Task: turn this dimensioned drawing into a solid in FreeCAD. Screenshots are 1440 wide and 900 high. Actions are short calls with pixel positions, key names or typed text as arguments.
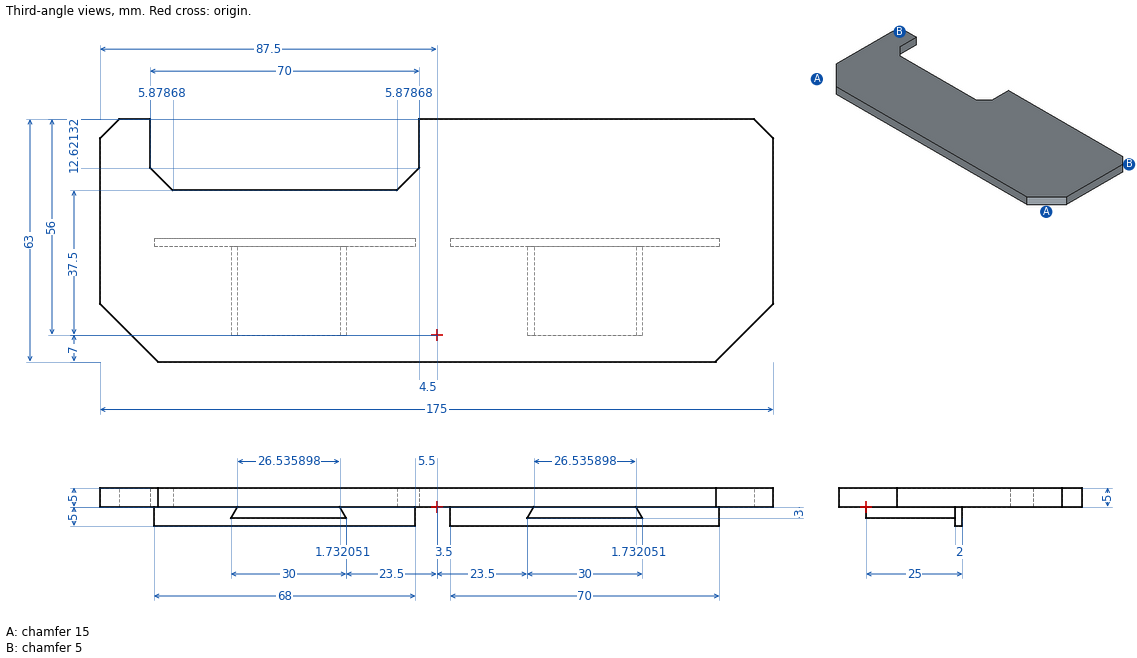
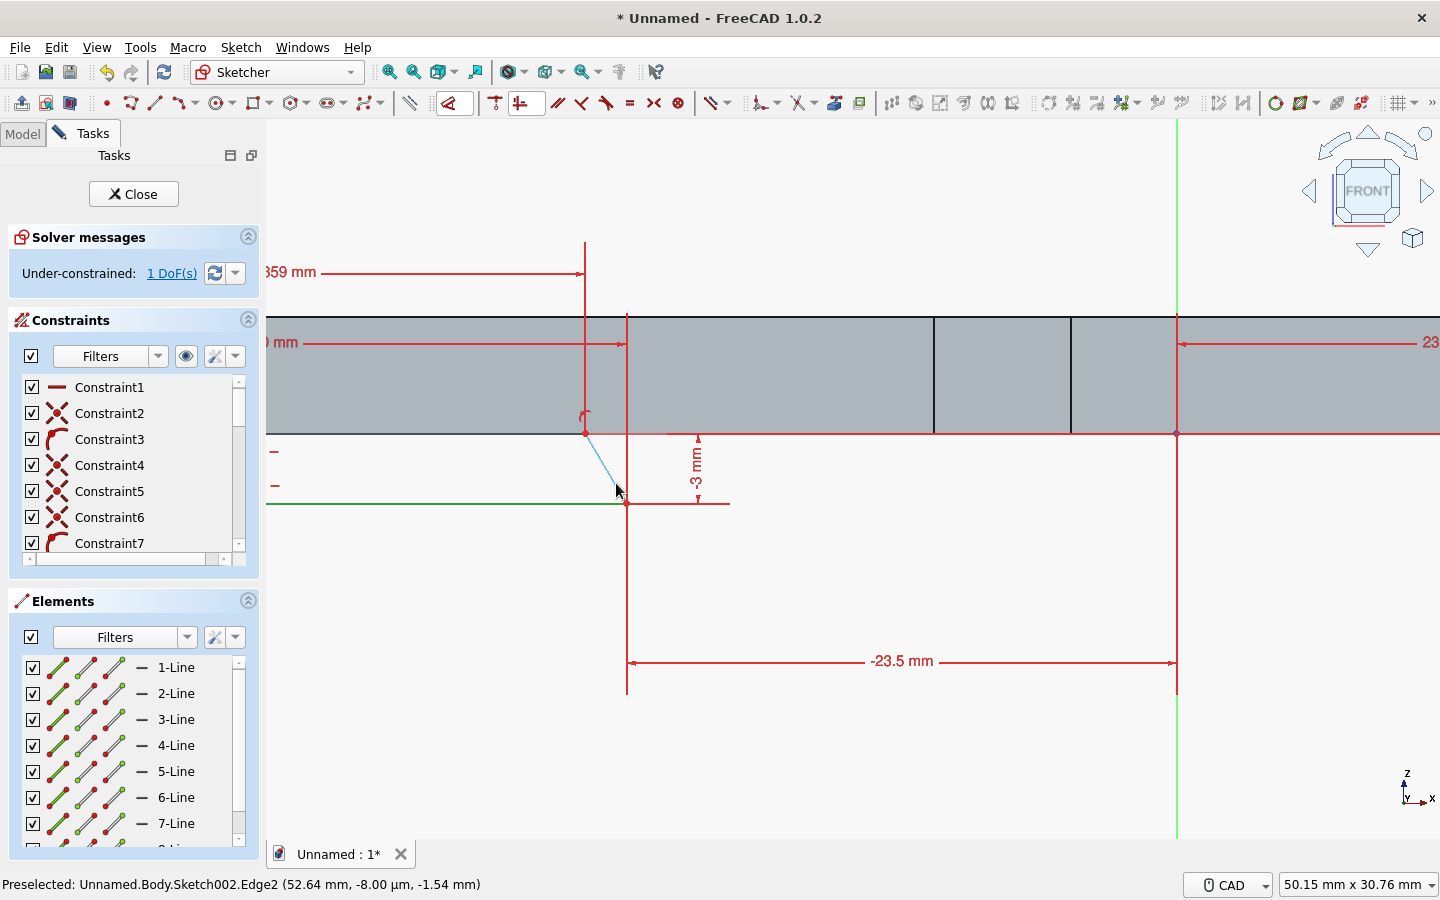
click(614, 483)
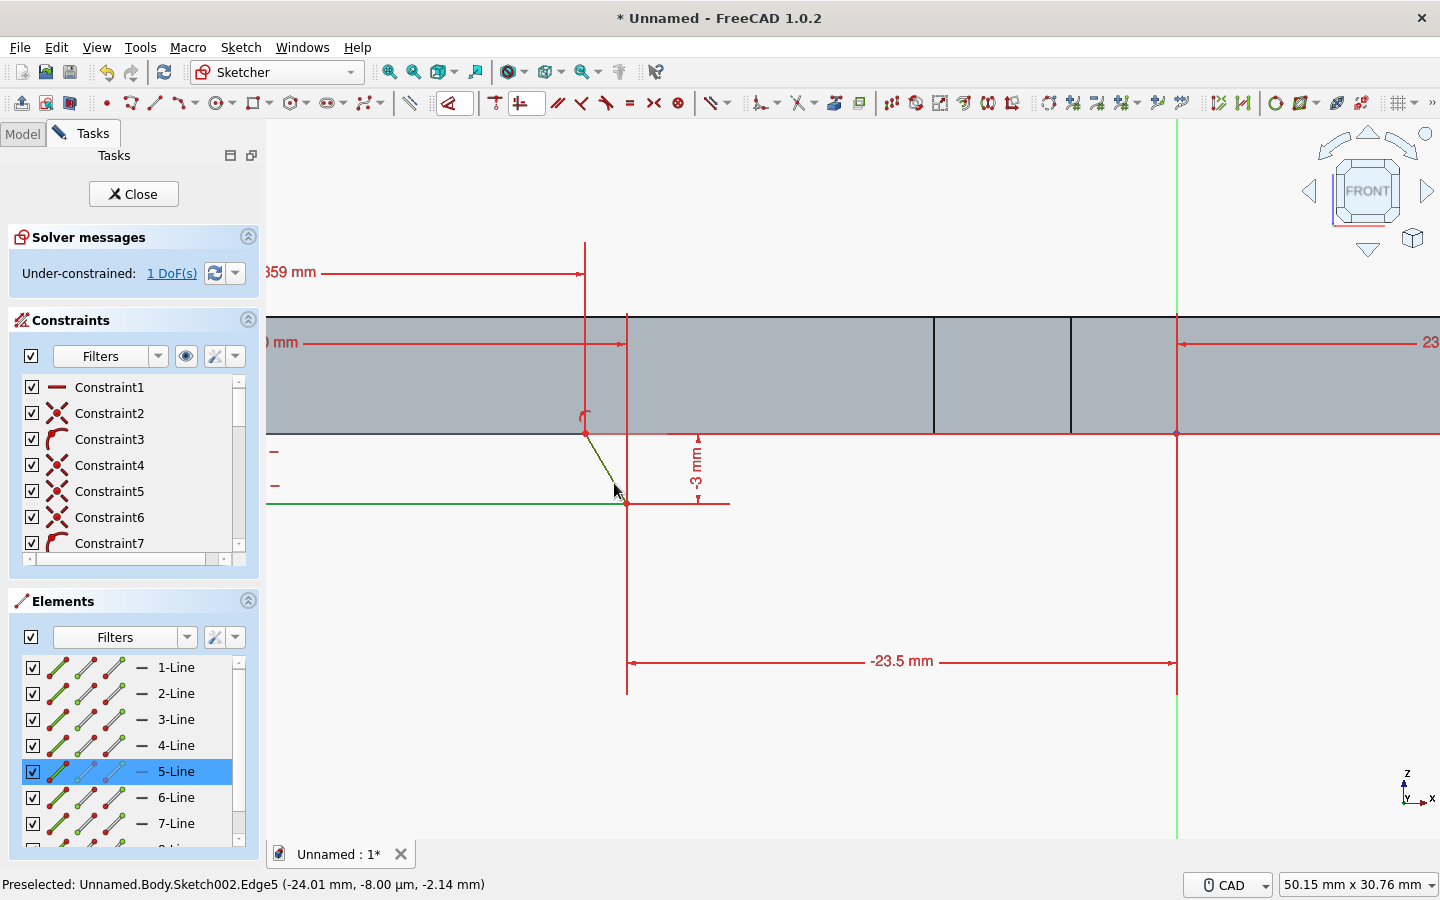
click(468, 104)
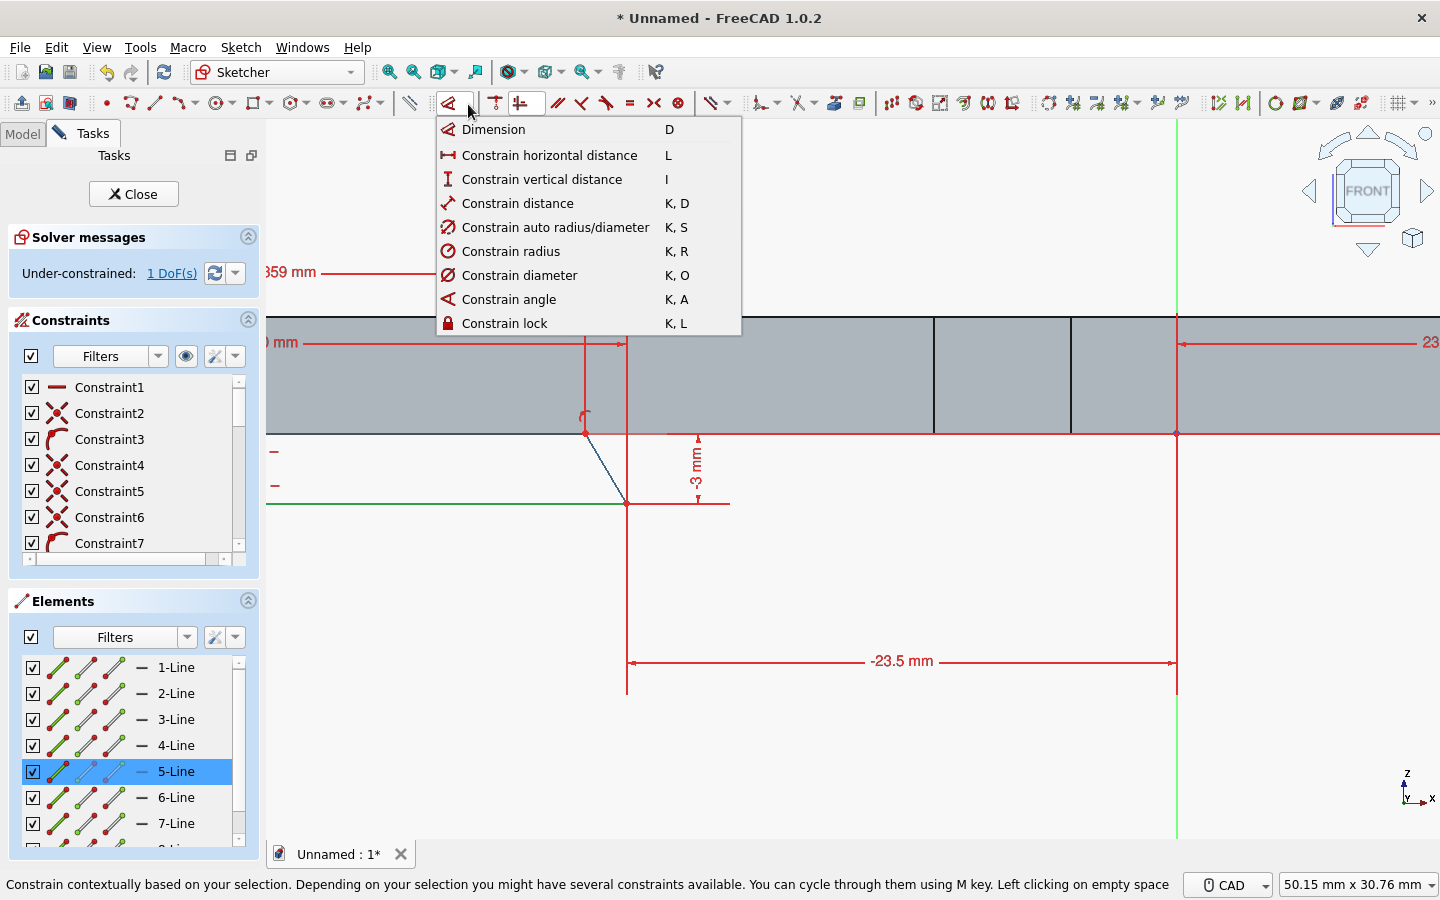
click(589, 155)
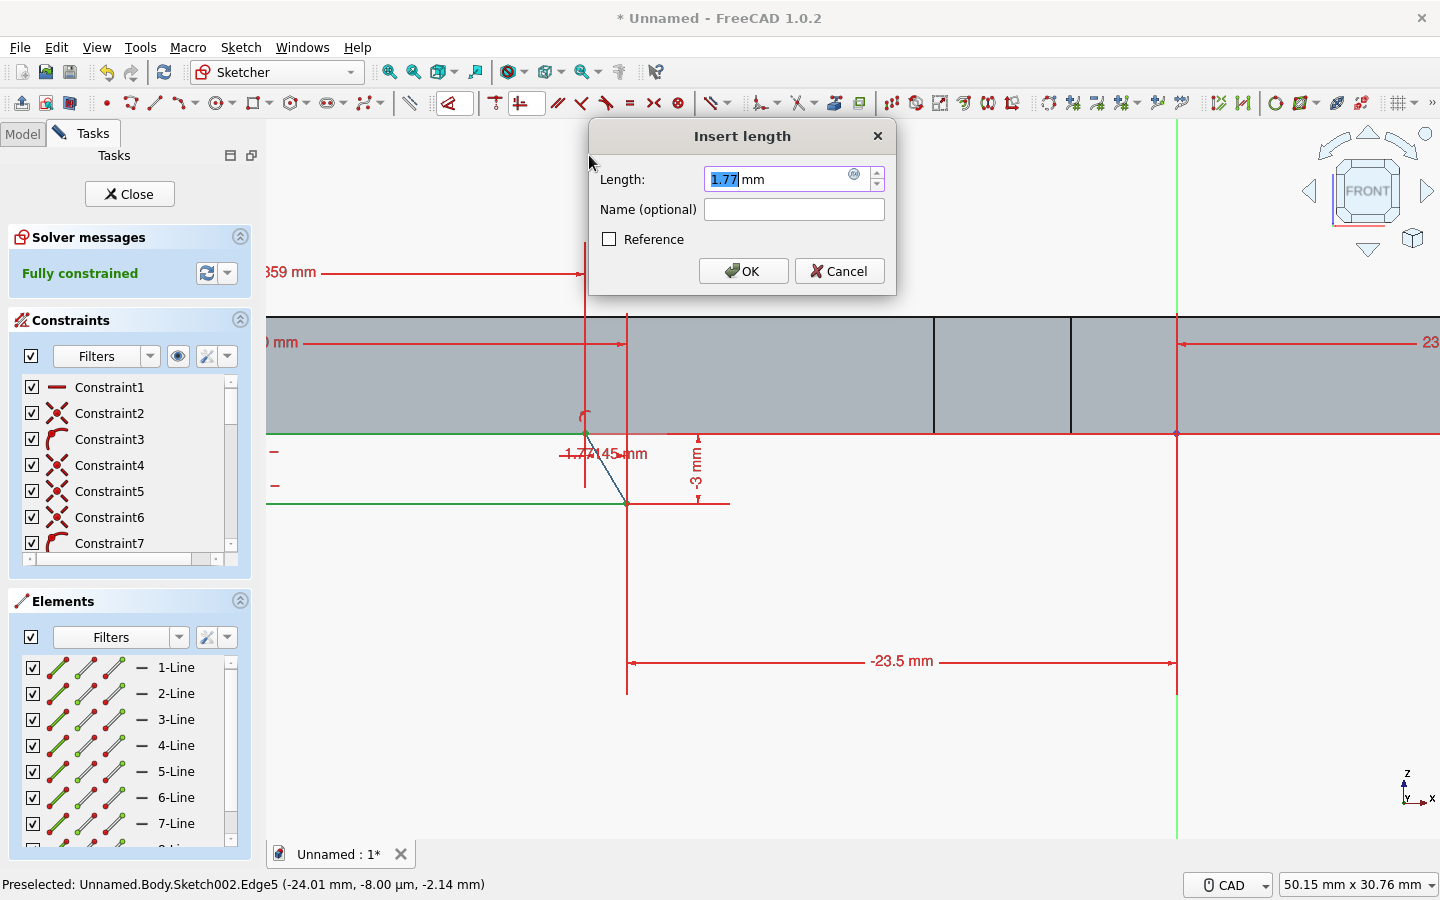
text(1.732051)
key(Return)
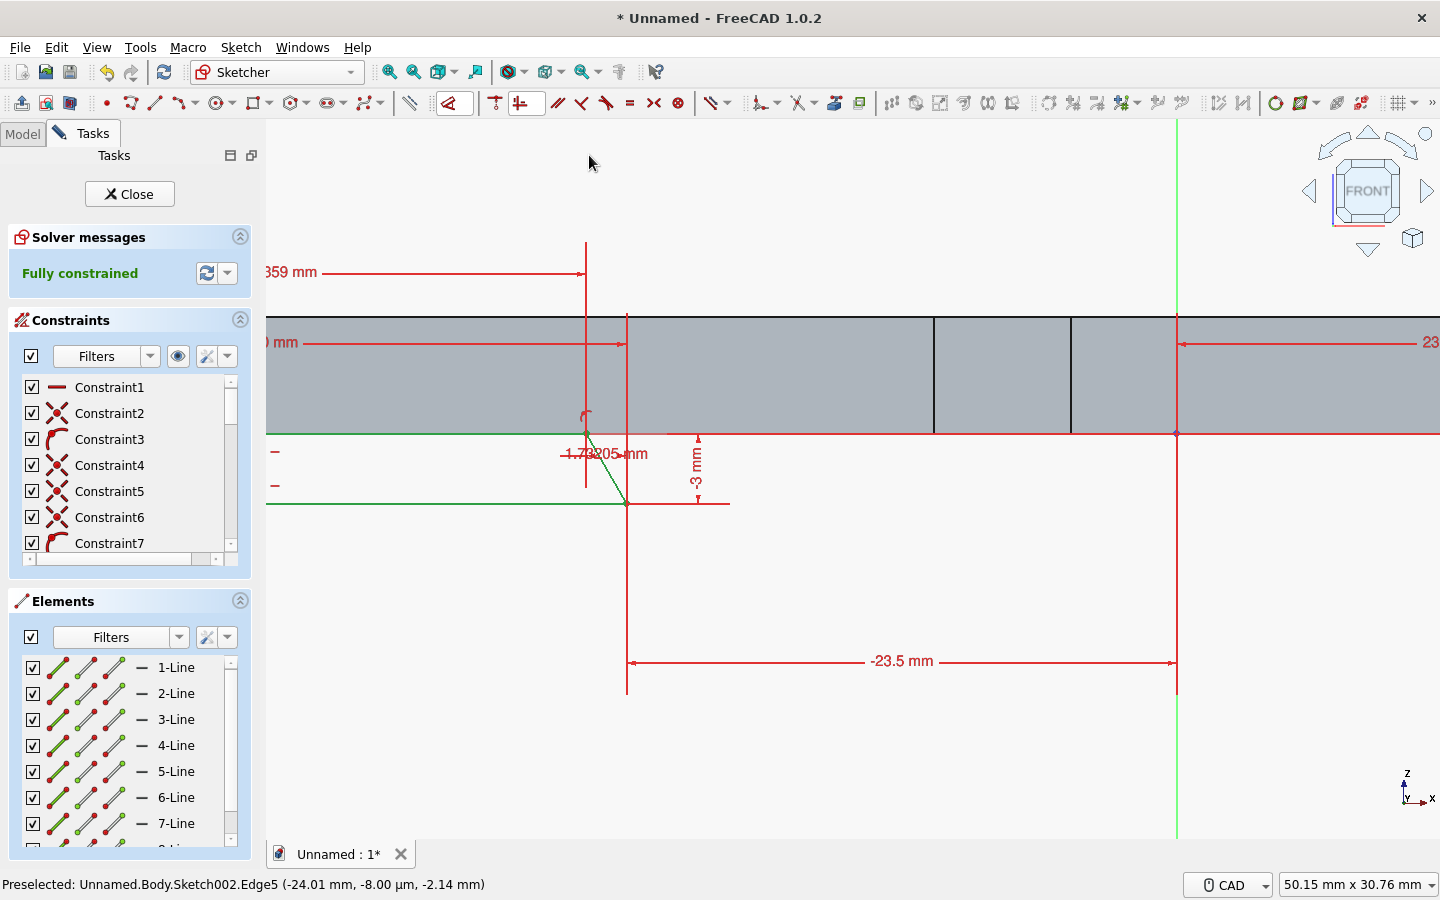
click(130, 194)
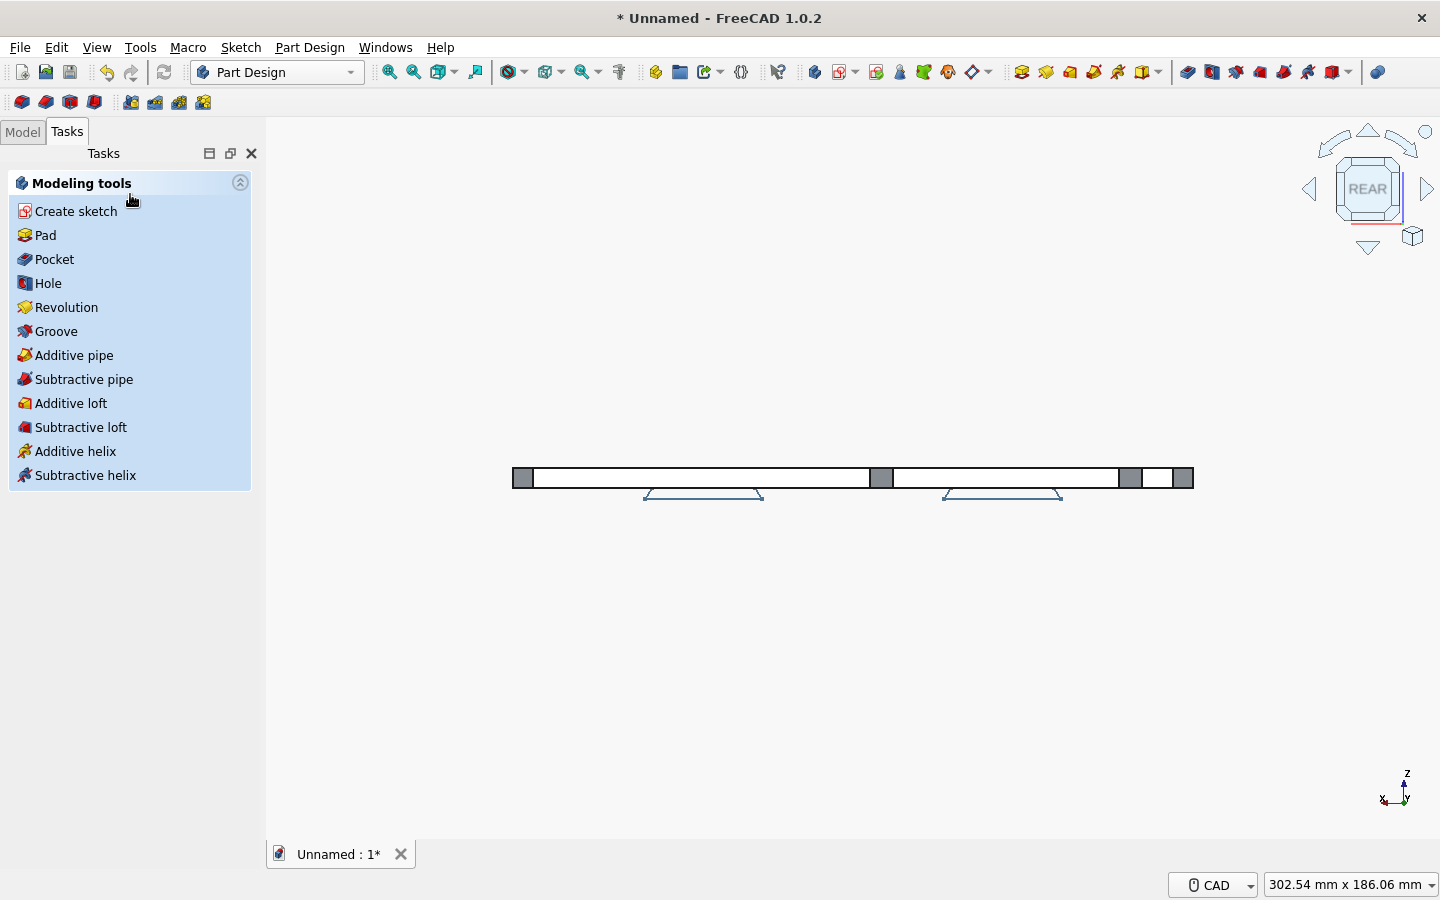
click(1022, 72)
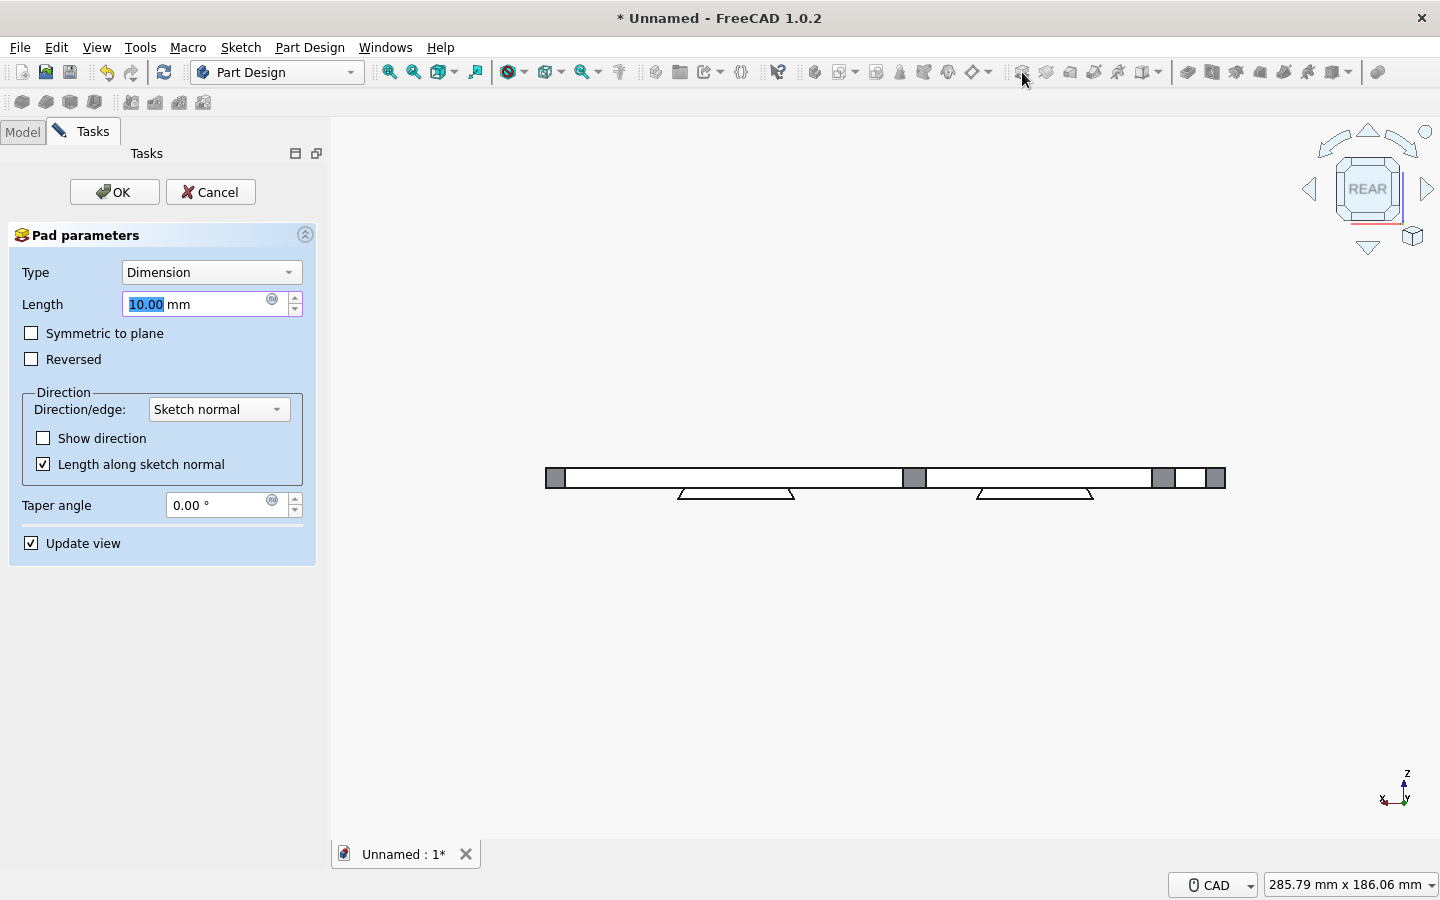
text(25)
key(Tab)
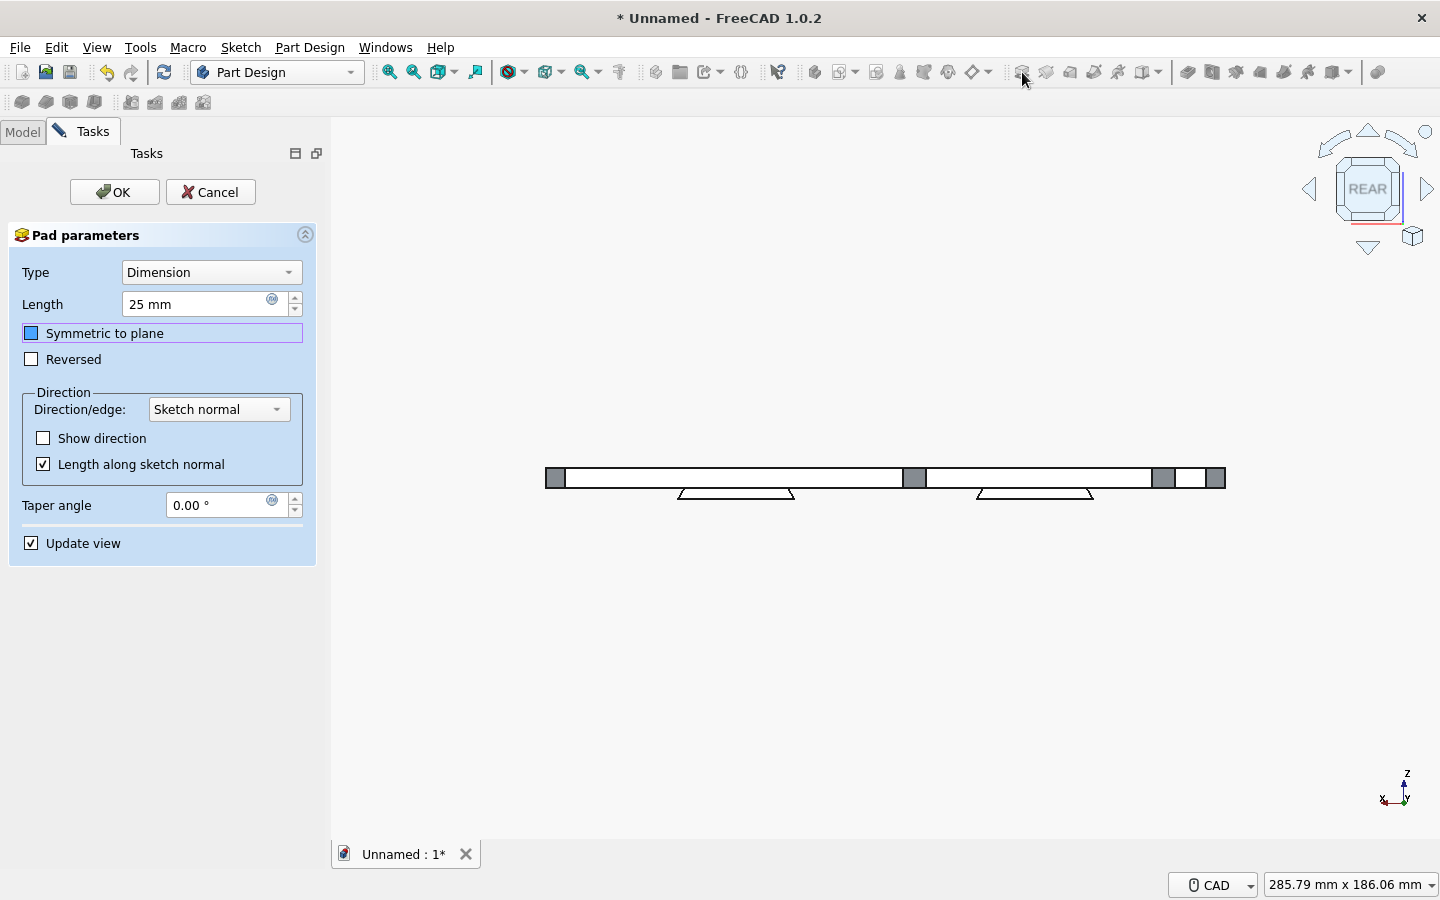
click(30, 359)